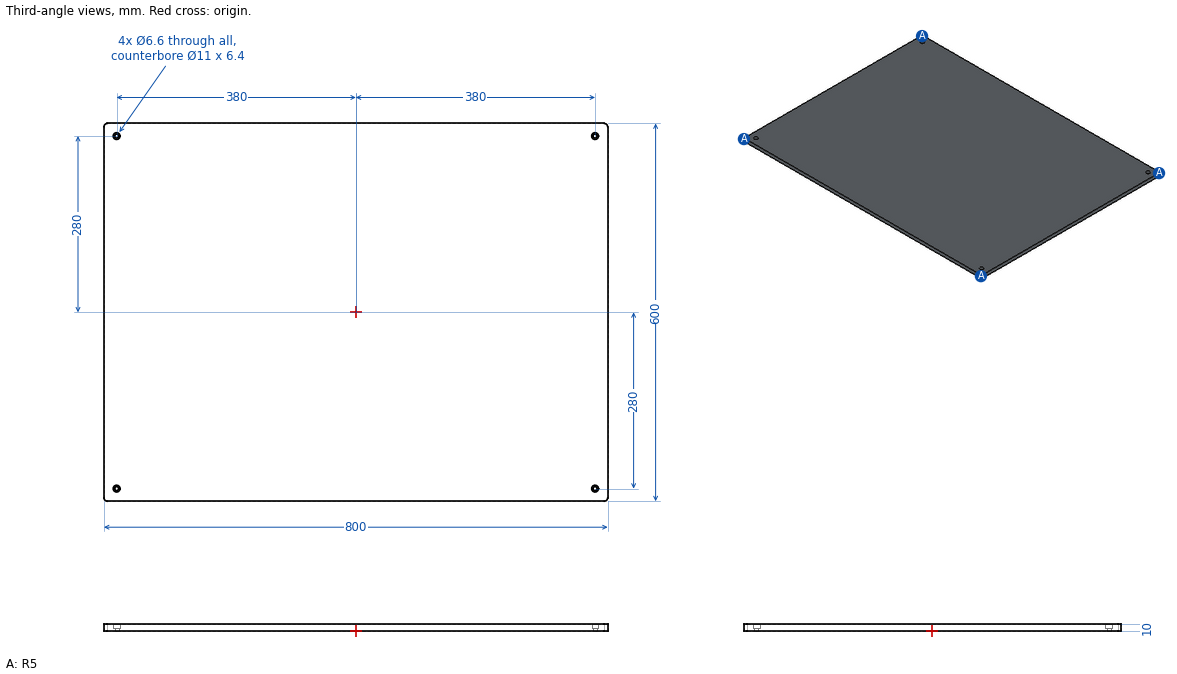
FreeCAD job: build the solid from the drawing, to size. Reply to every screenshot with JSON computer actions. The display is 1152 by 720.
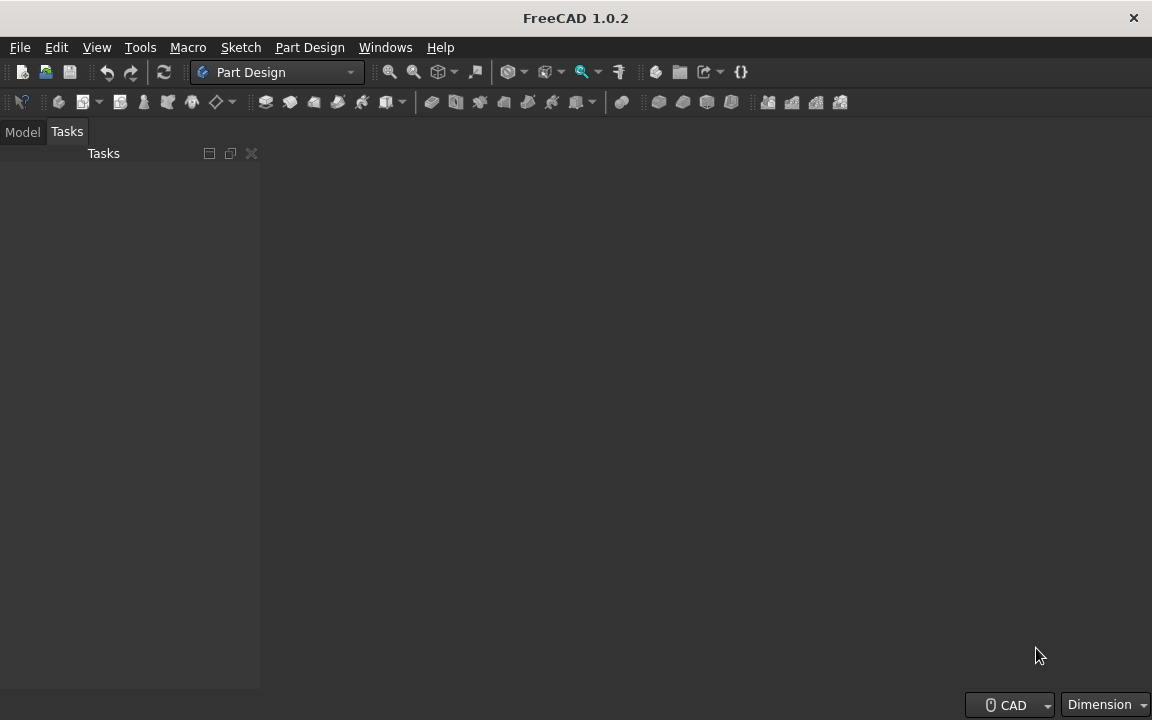
{"action": "key", "text": "ctrl+n"}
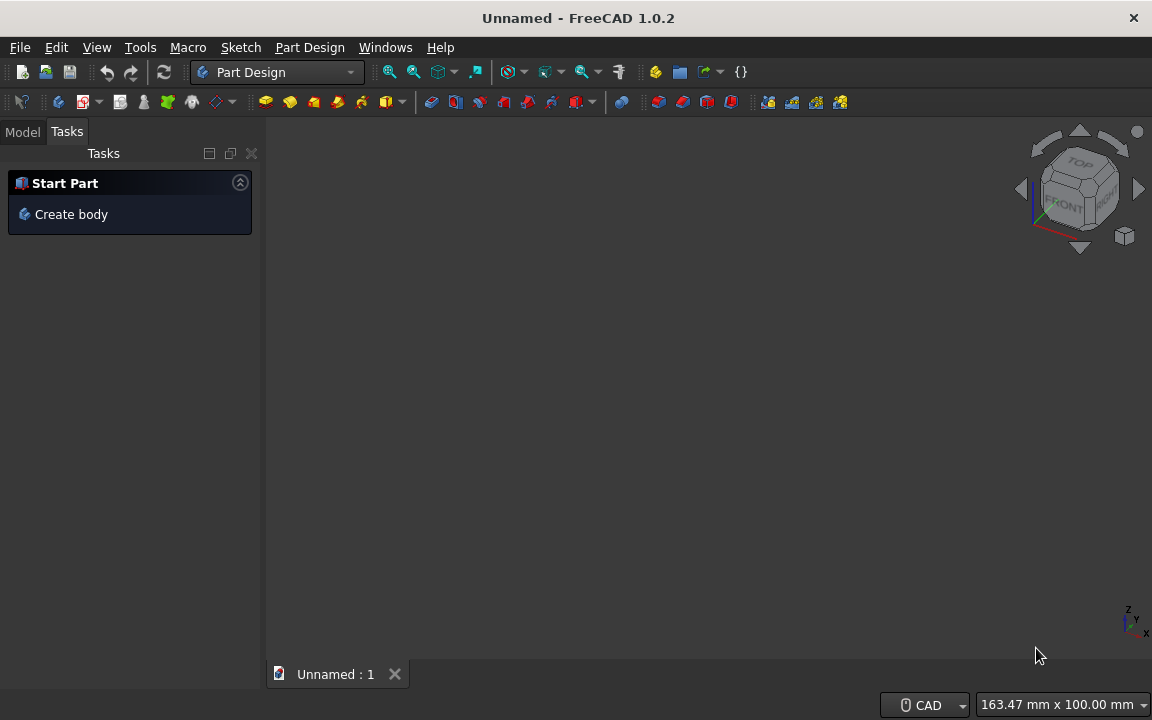
{"action": "left_click", "coordinate": [84, 102]}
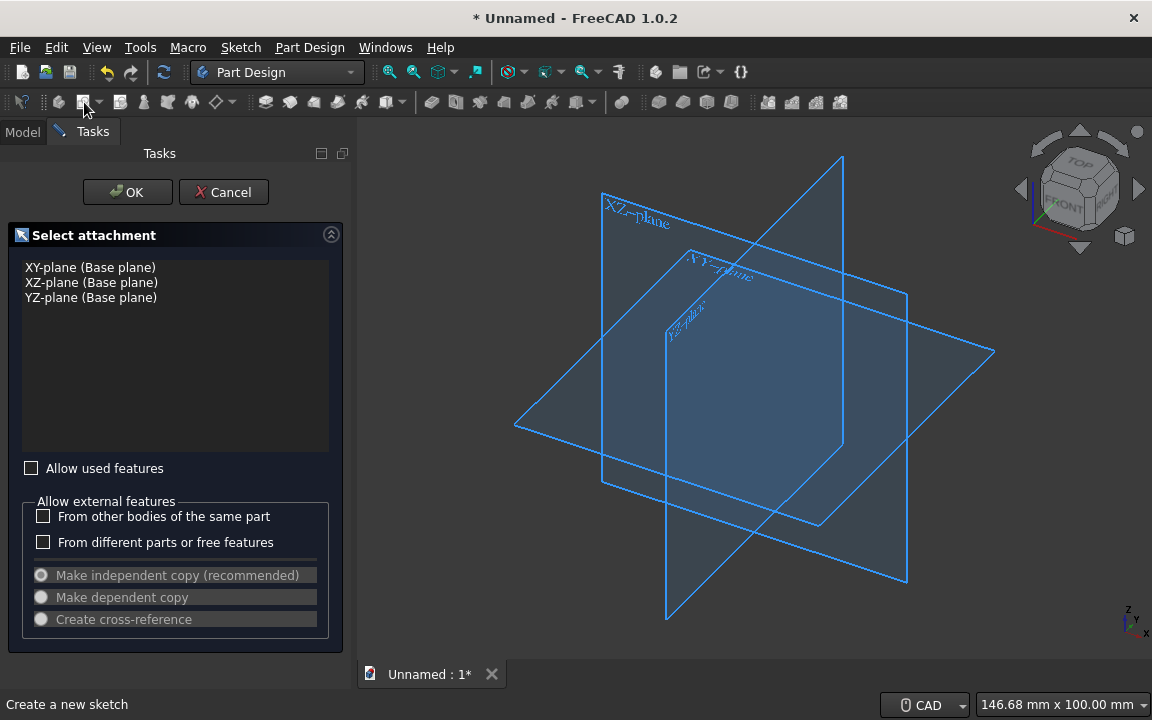
{"action": "left_click", "coordinate": [82, 268]}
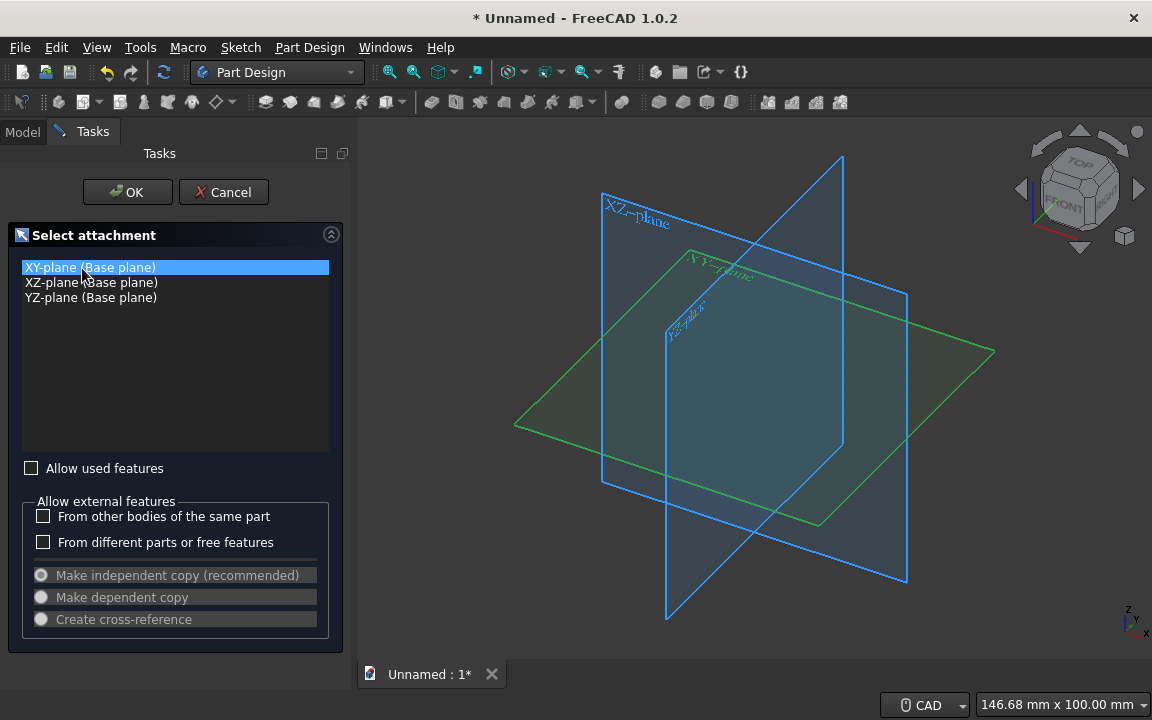
{"action": "left_click", "coordinate": [128, 192]}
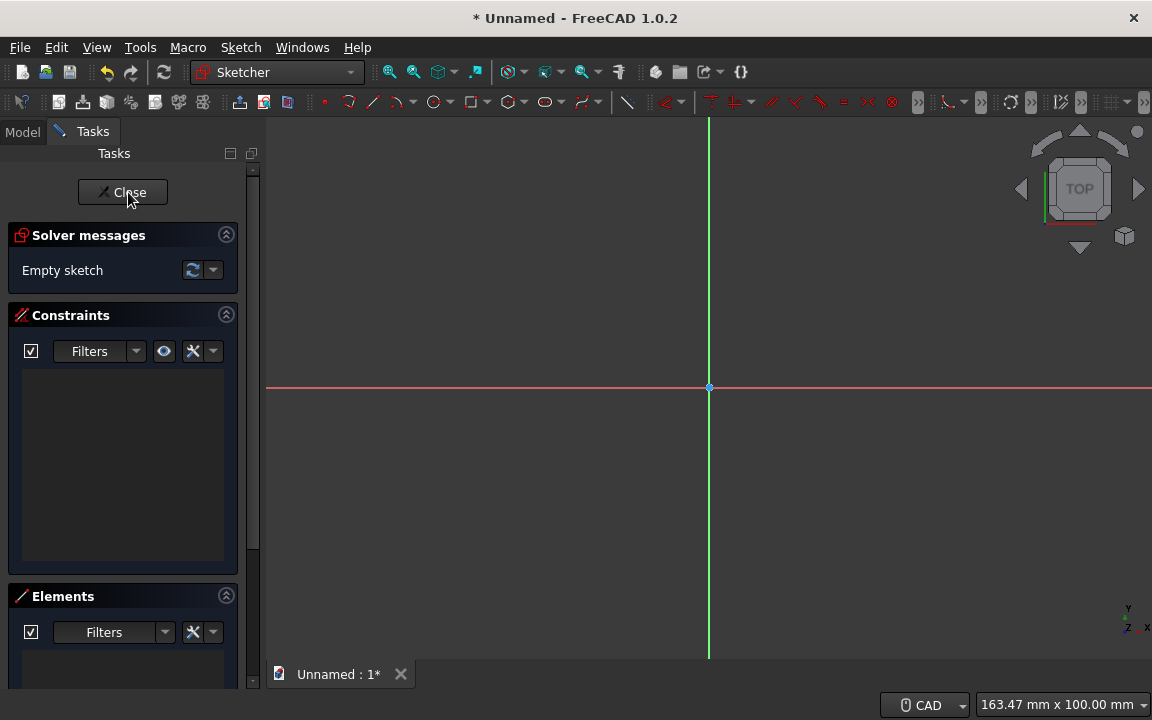
{"action": "scroll", "coordinate": [632, 388], "scroll_direction": "down", "scroll_amount": 11}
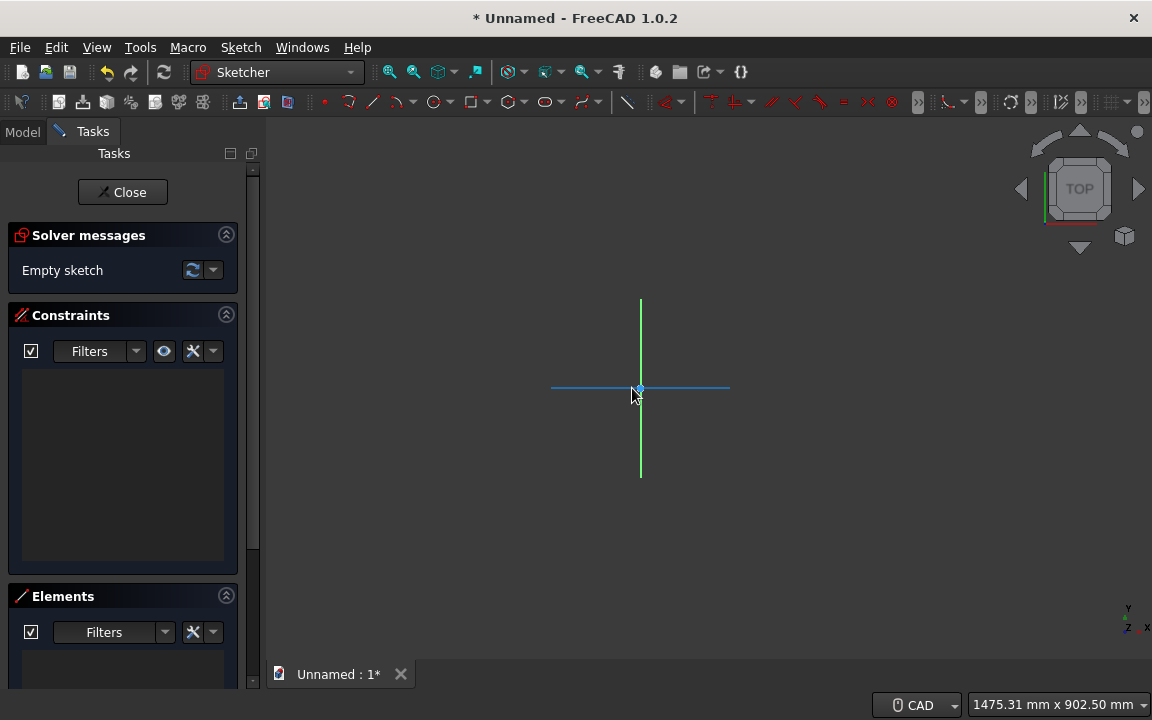
{"action": "key", "text": "g v"}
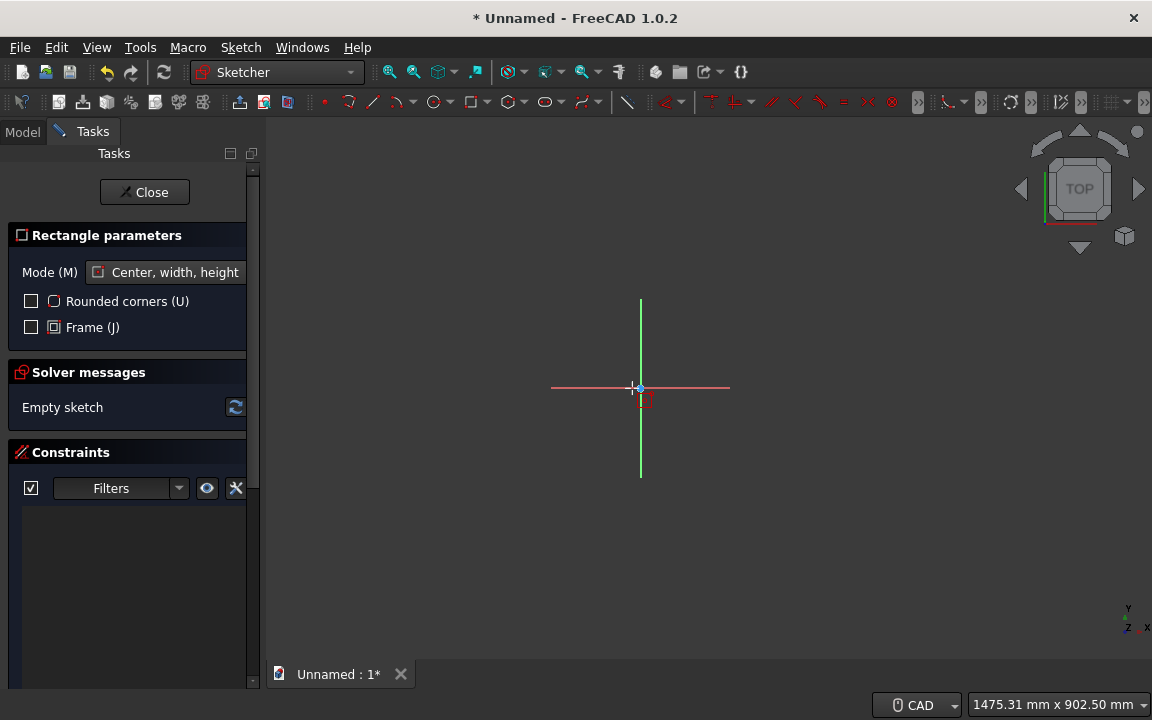
{"action": "left_click", "coordinate": [641, 388]}
{"action": "mouse_move", "coordinate": [881, 208]}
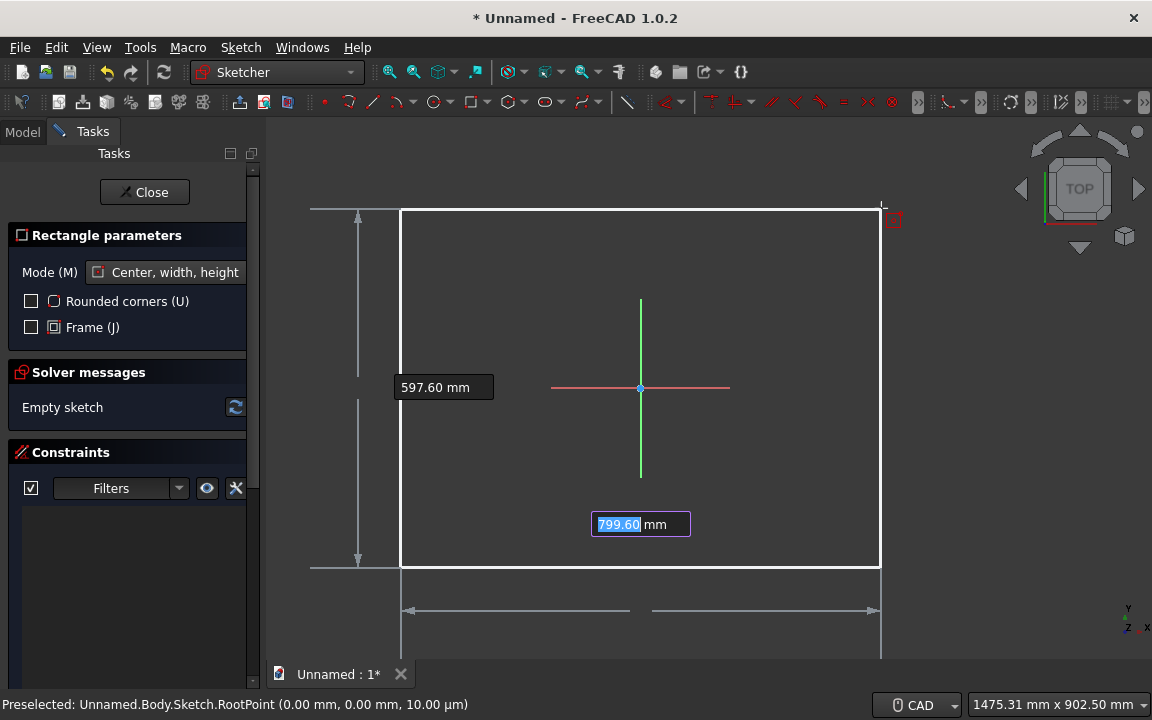
{"action": "type", "text": "800"}
{"action": "key", "text": "Tab"}
{"action": "type", "text": "600"}
{"action": "key", "text": "Return"}
{"action": "key", "text": "Escape"}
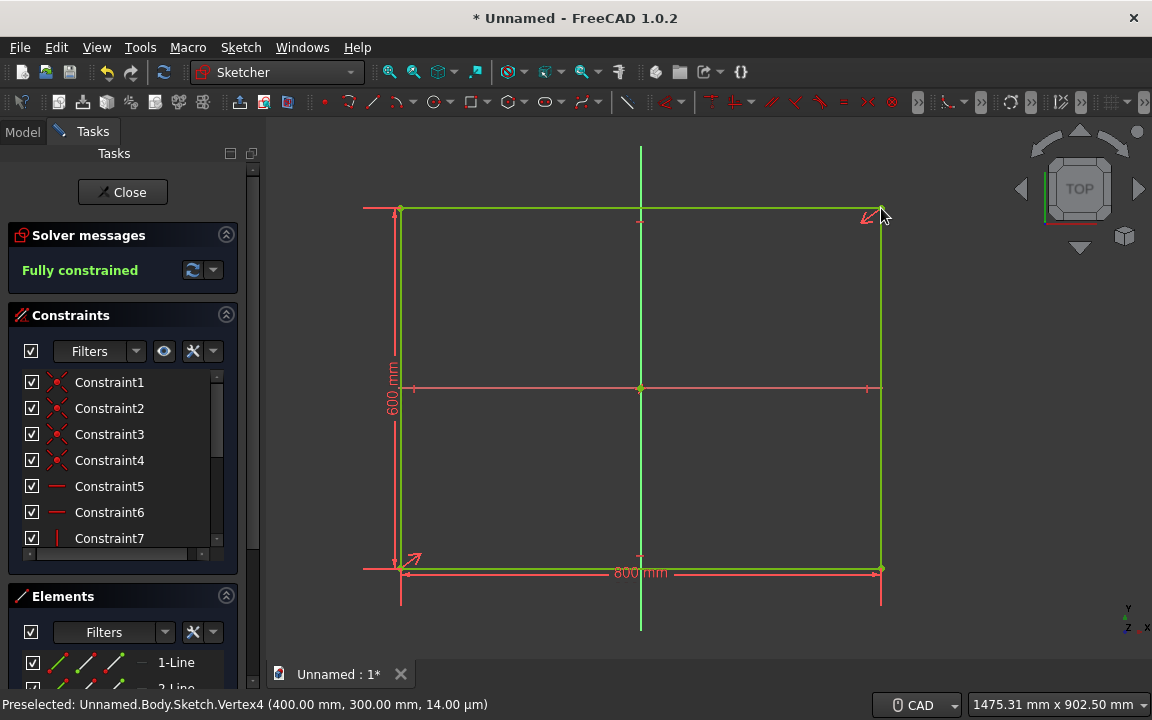
{"action": "left_click", "coordinate": [123, 192]}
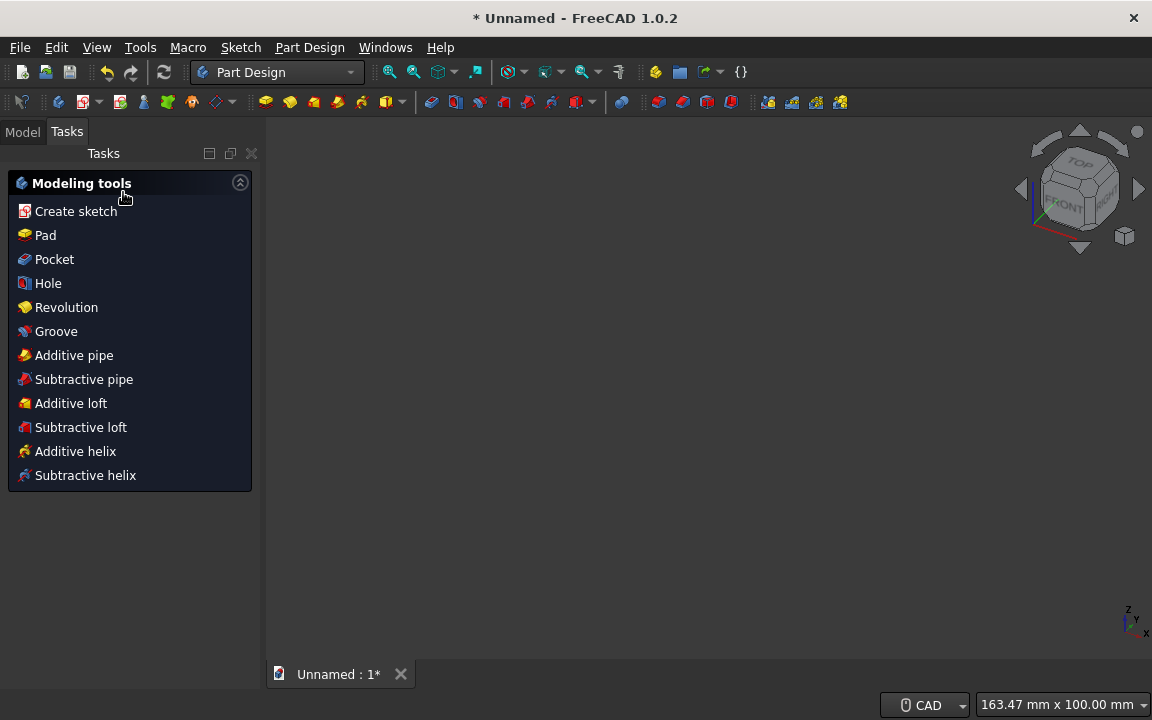
{"action": "left_click", "coordinate": [266, 102]}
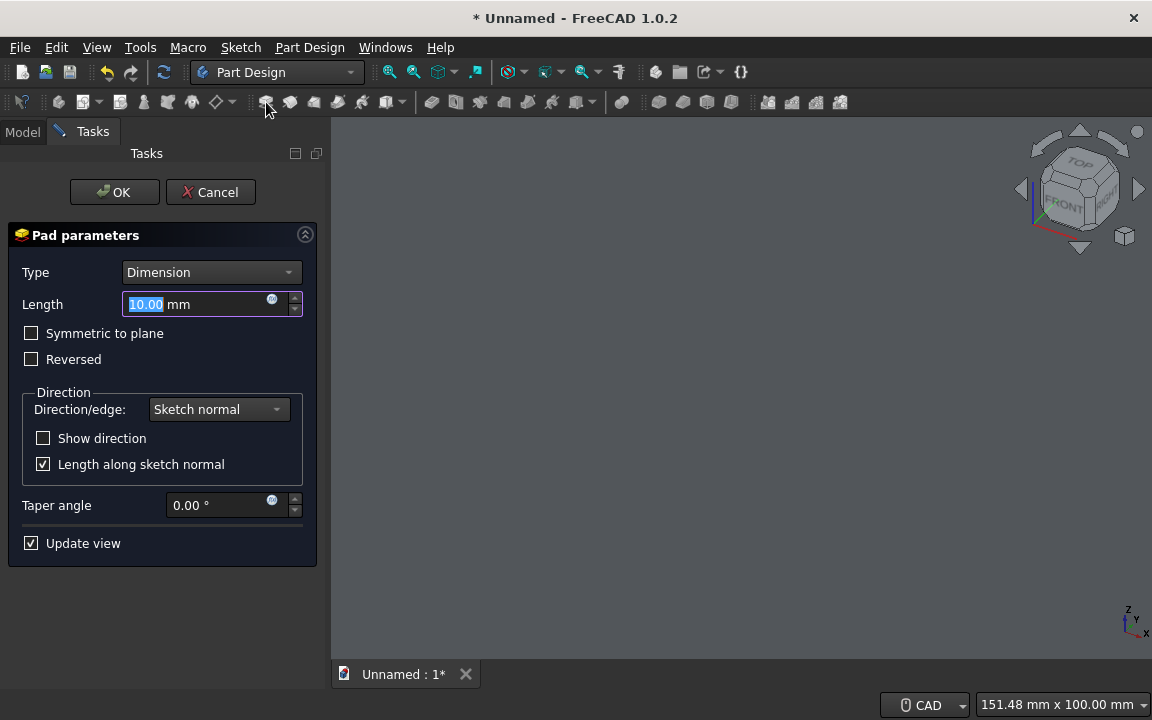
{"action": "type", "text": "10"}
{"action": "key", "text": "Tab"}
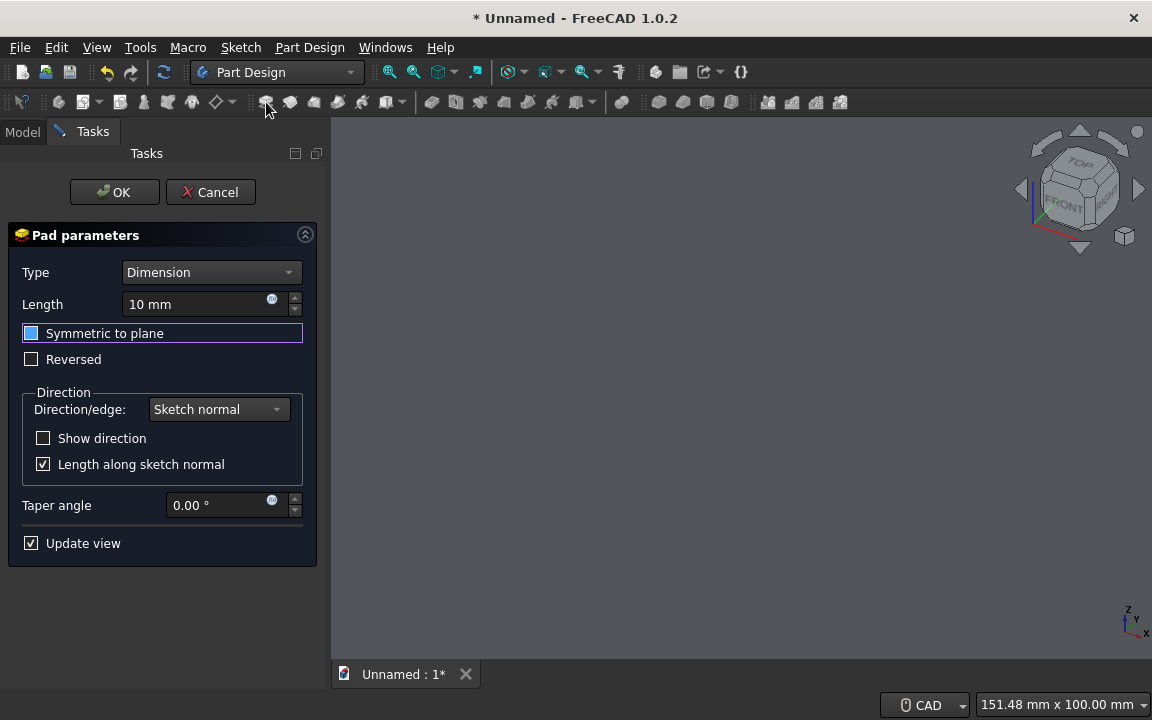
{"action": "left_click", "coordinate": [115, 192]}